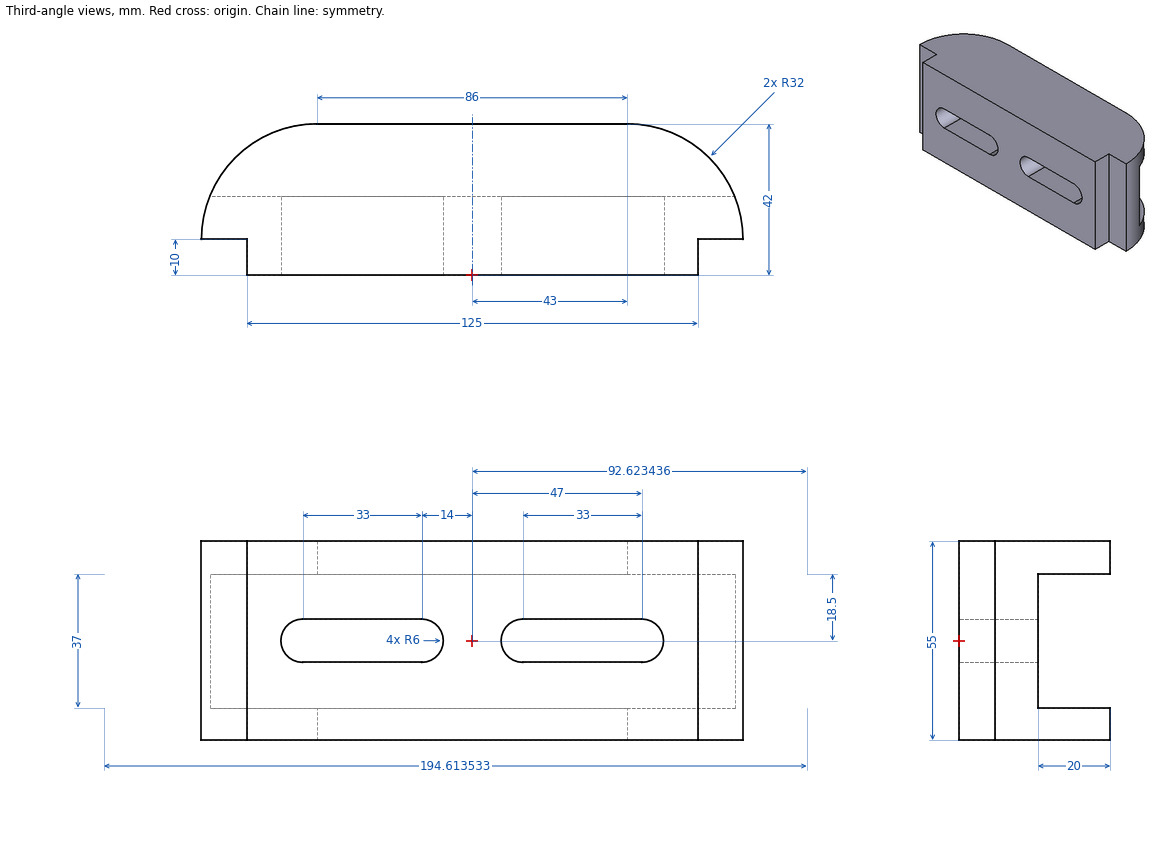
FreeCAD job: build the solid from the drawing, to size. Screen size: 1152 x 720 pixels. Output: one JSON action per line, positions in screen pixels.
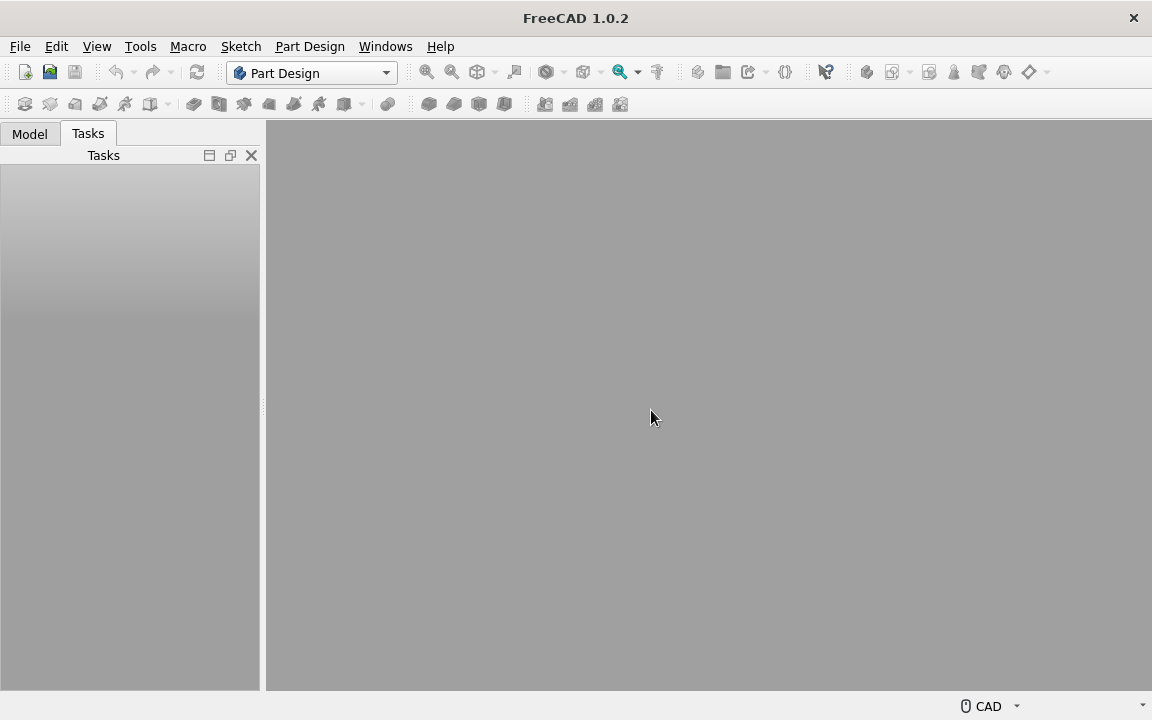
{"action": "left_click", "coordinate": [25, 72]}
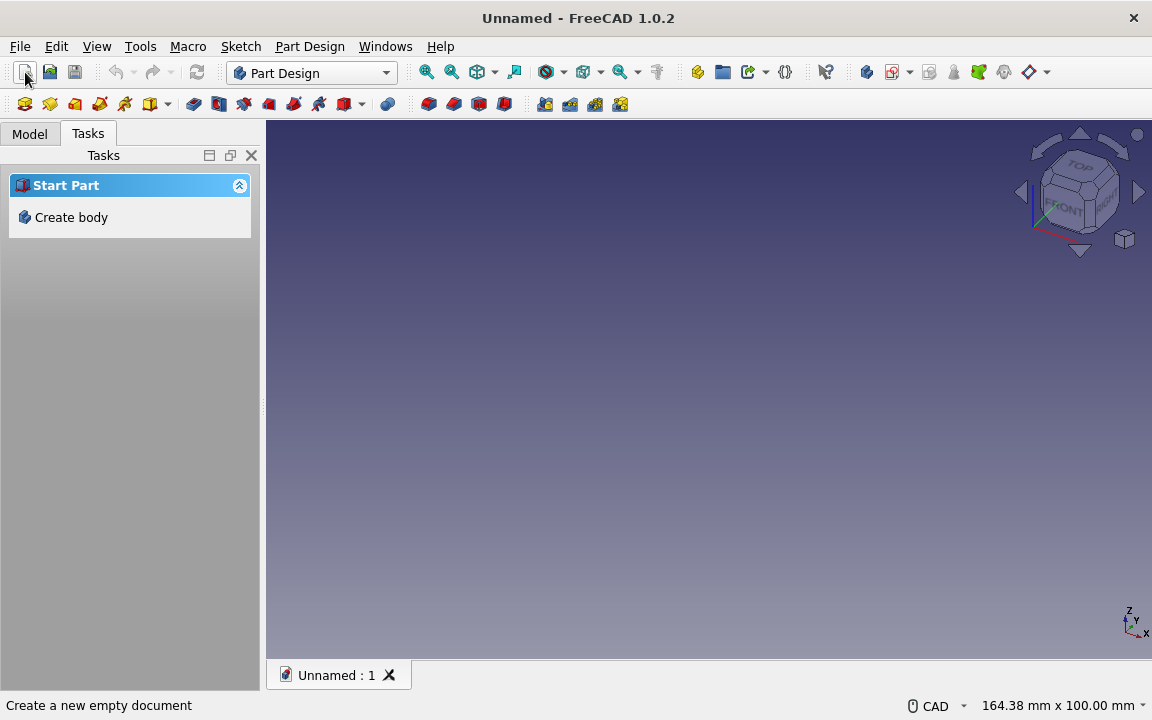
{"action": "left_click", "coordinate": [892, 72]}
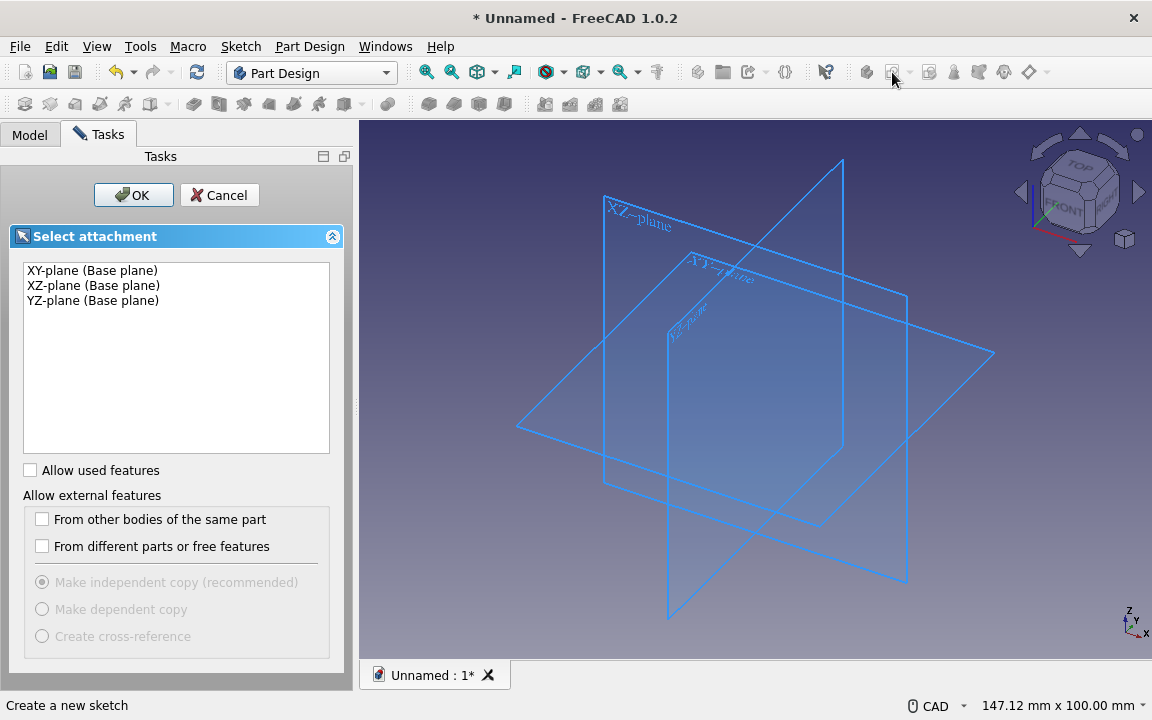
{"action": "left_click", "coordinate": [84, 270]}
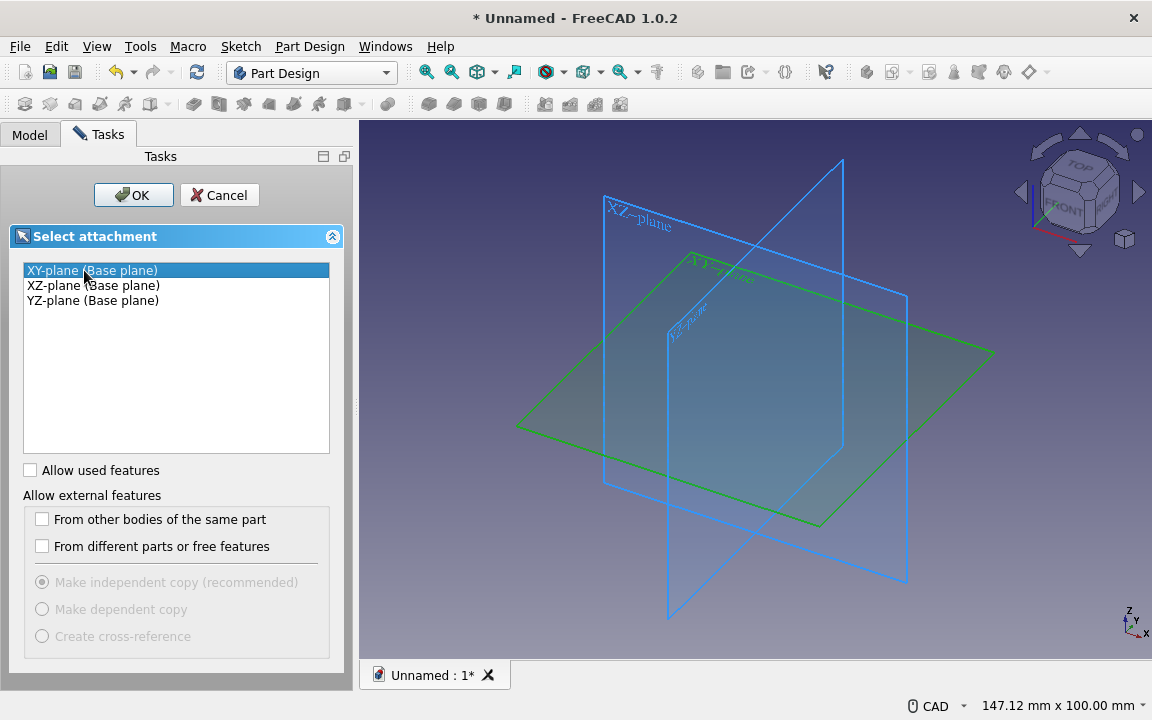
{"action": "left_click", "coordinate": [134, 195]}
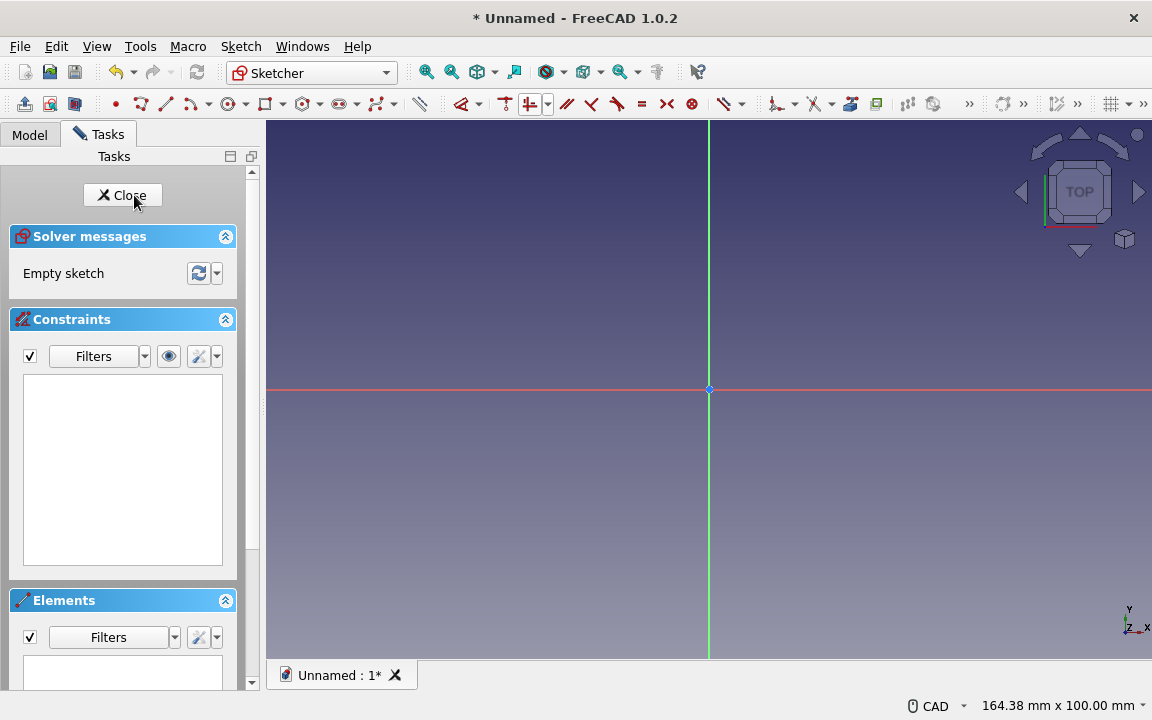
{"action": "scroll", "coordinate": [557, 527], "scroll_direction": "down", "scroll_amount": 3}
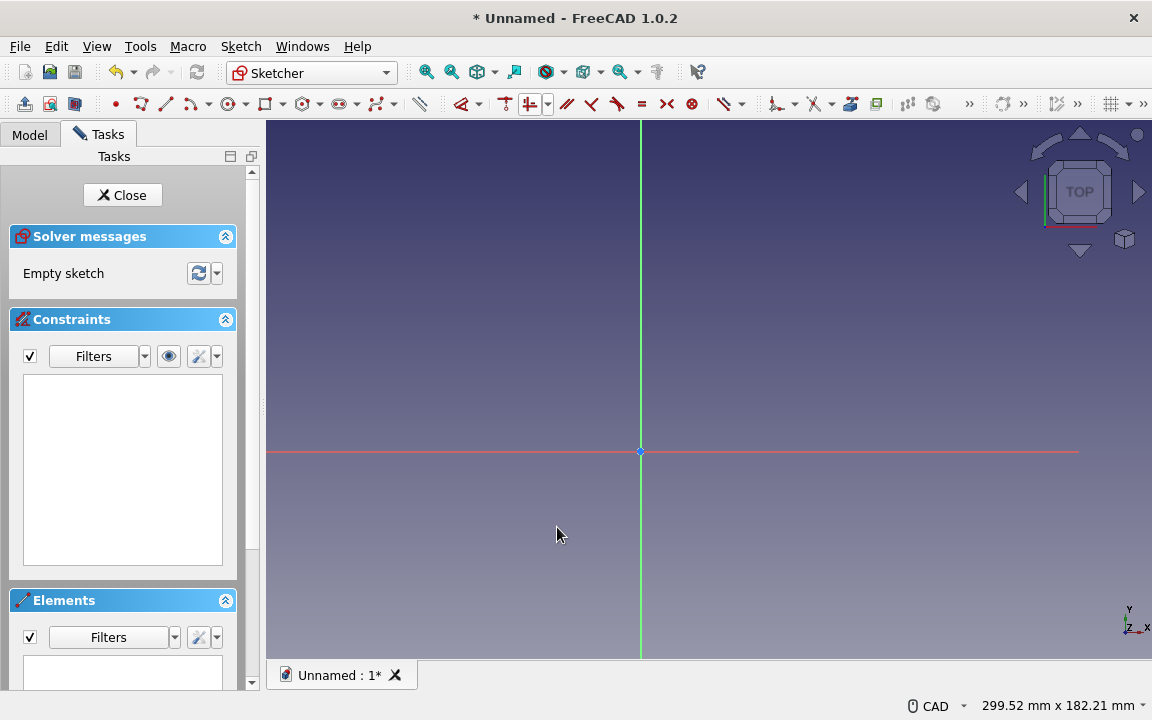
{"action": "left_click", "coordinate": [166, 104]}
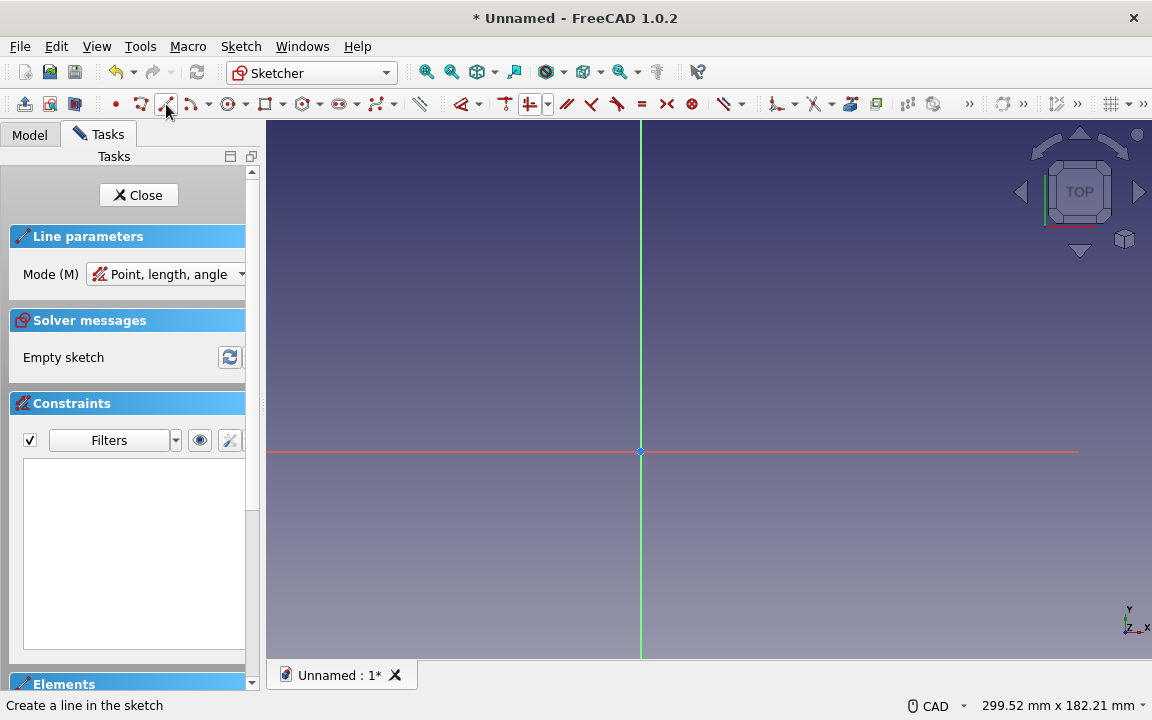
{"action": "left_click", "coordinate": [768, 328]}
{"action": "left_click", "coordinate": [513, 328]}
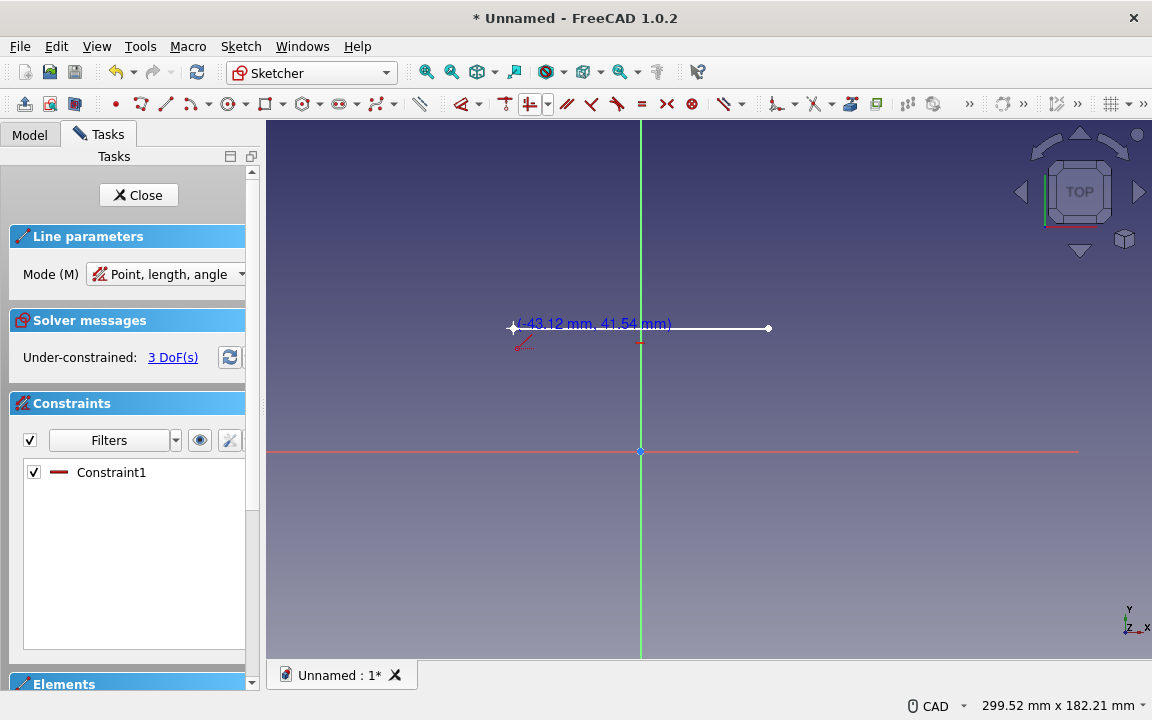
{"action": "left_click", "coordinate": [141, 104]}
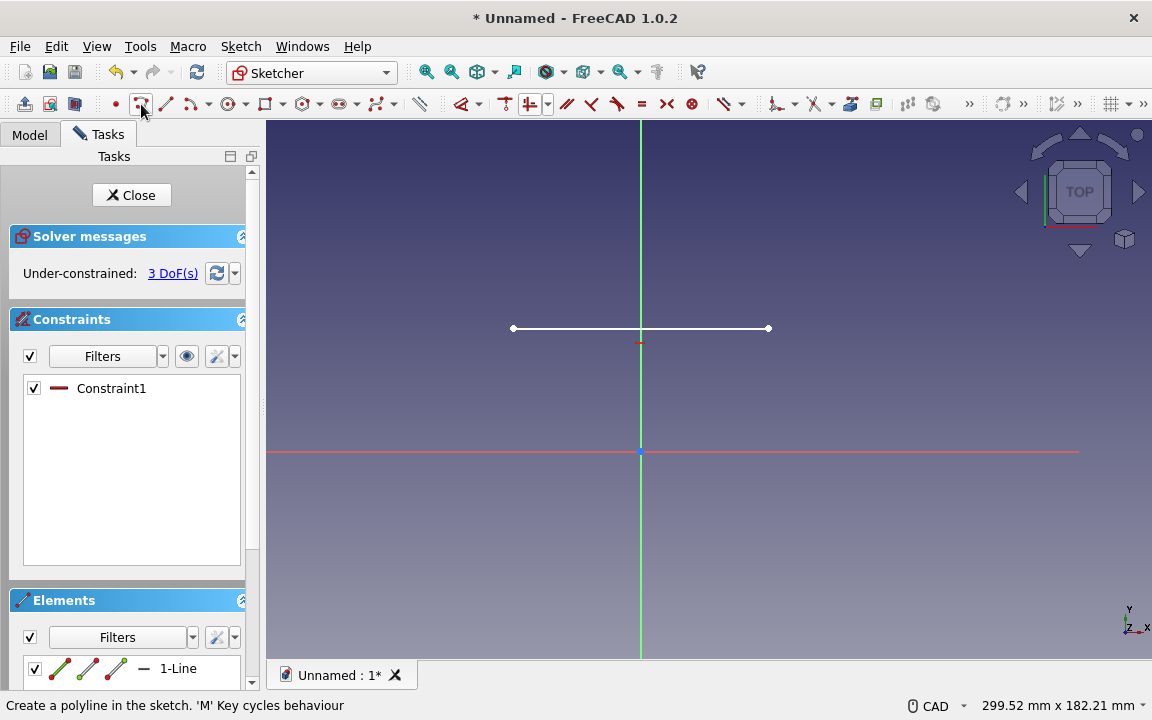
{"action": "left_click", "coordinate": [419, 422]}
{"action": "left_click", "coordinate": [456, 422]}
{"action": "left_click", "coordinate": [456, 452]}
{"action": "left_click", "coordinate": [825, 443]}
{"action": "left_click", "coordinate": [825, 422]}
{"action": "left_click", "coordinate": [862, 422]}
{"action": "right_click", "coordinate": [862, 422]}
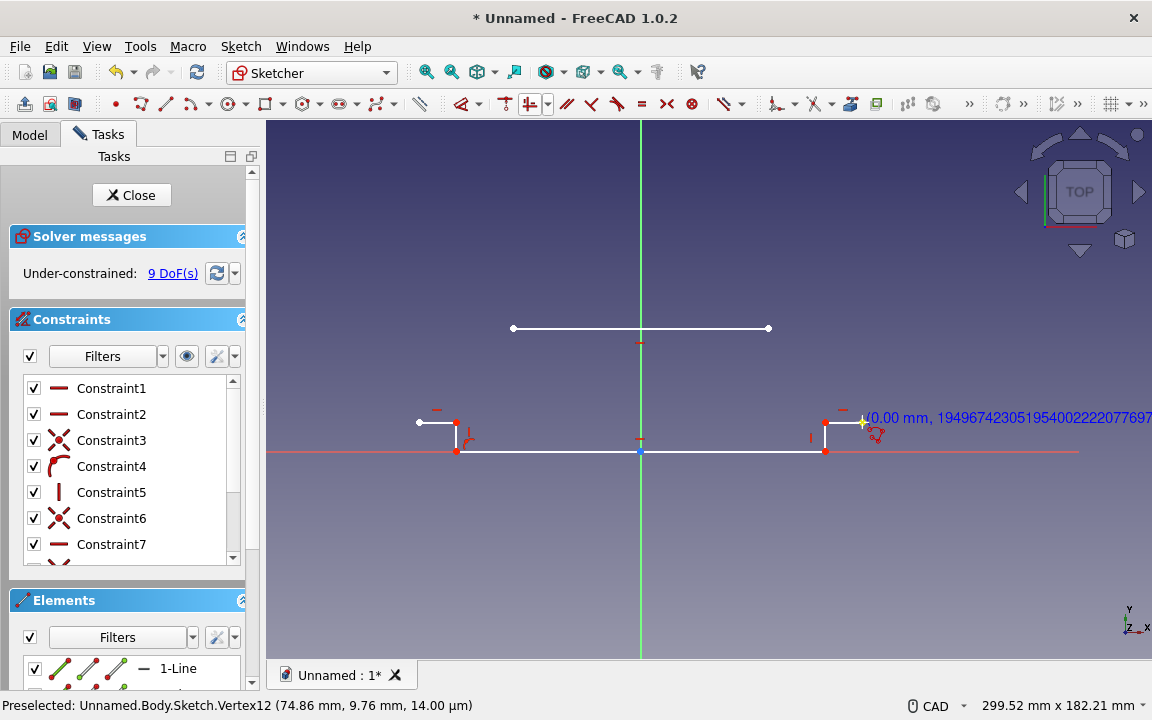
{"action": "left_click", "coordinate": [208, 104]}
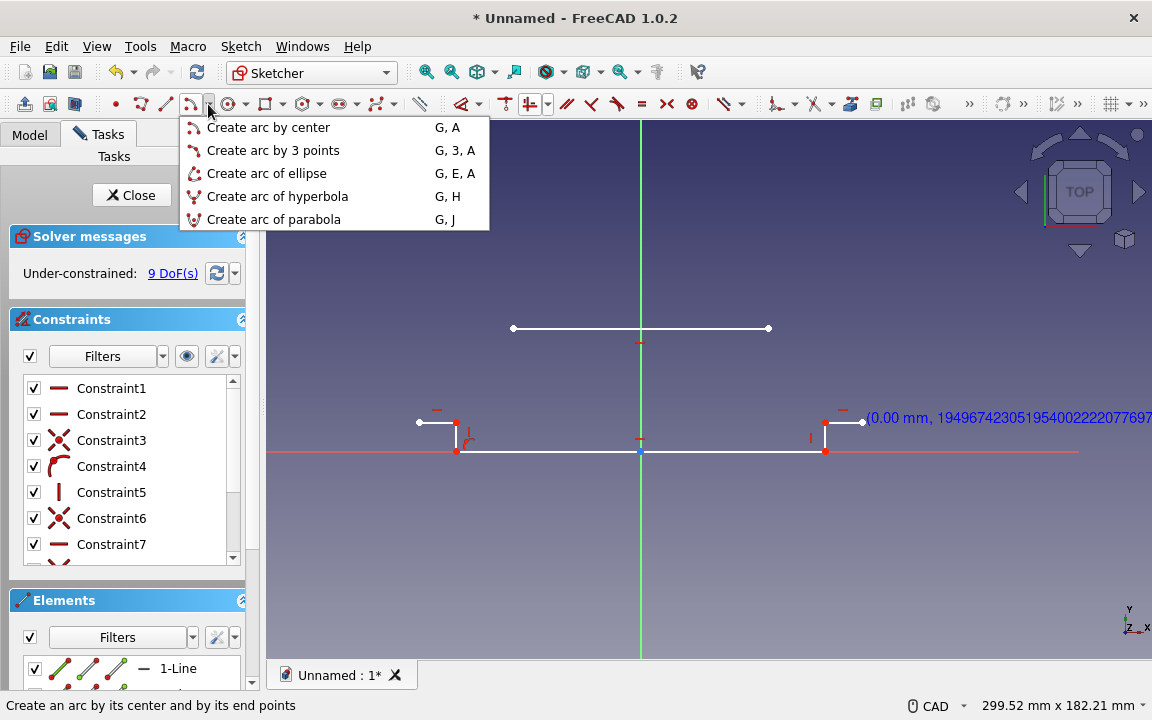
{"action": "left_click", "coordinate": [334, 150]}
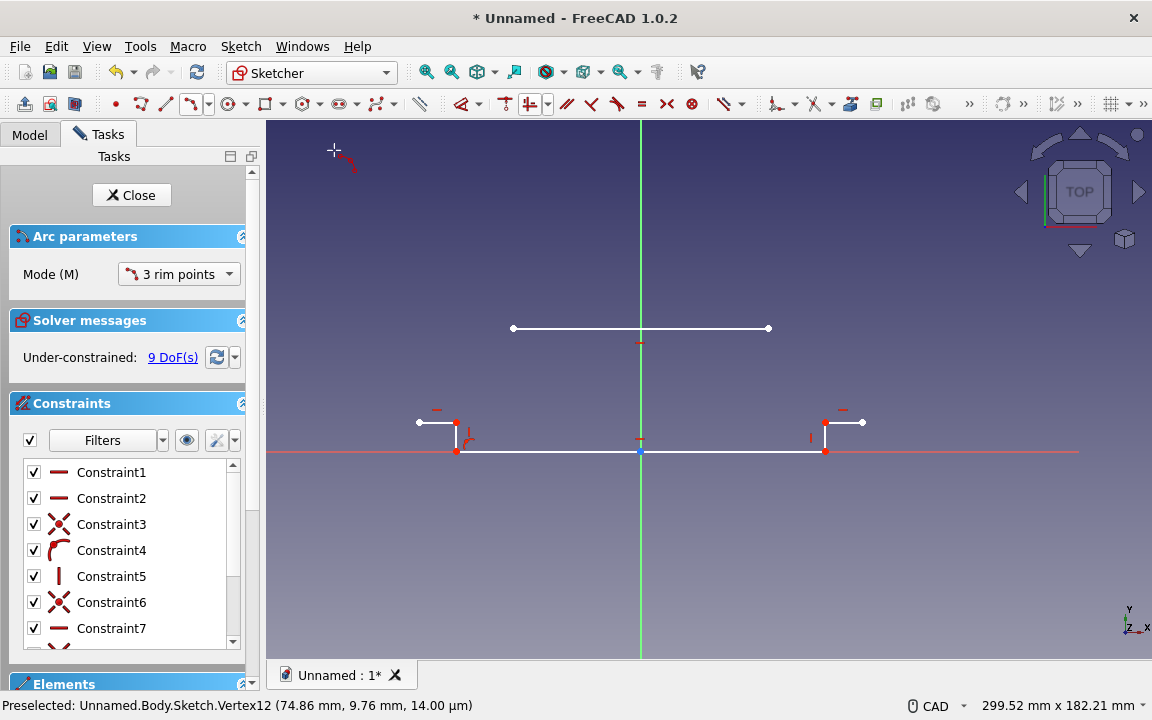
{"action": "left_click", "coordinate": [513, 329]}
{"action": "left_click", "coordinate": [419, 423]}
{"action": "left_click", "coordinate": [446, 355]}